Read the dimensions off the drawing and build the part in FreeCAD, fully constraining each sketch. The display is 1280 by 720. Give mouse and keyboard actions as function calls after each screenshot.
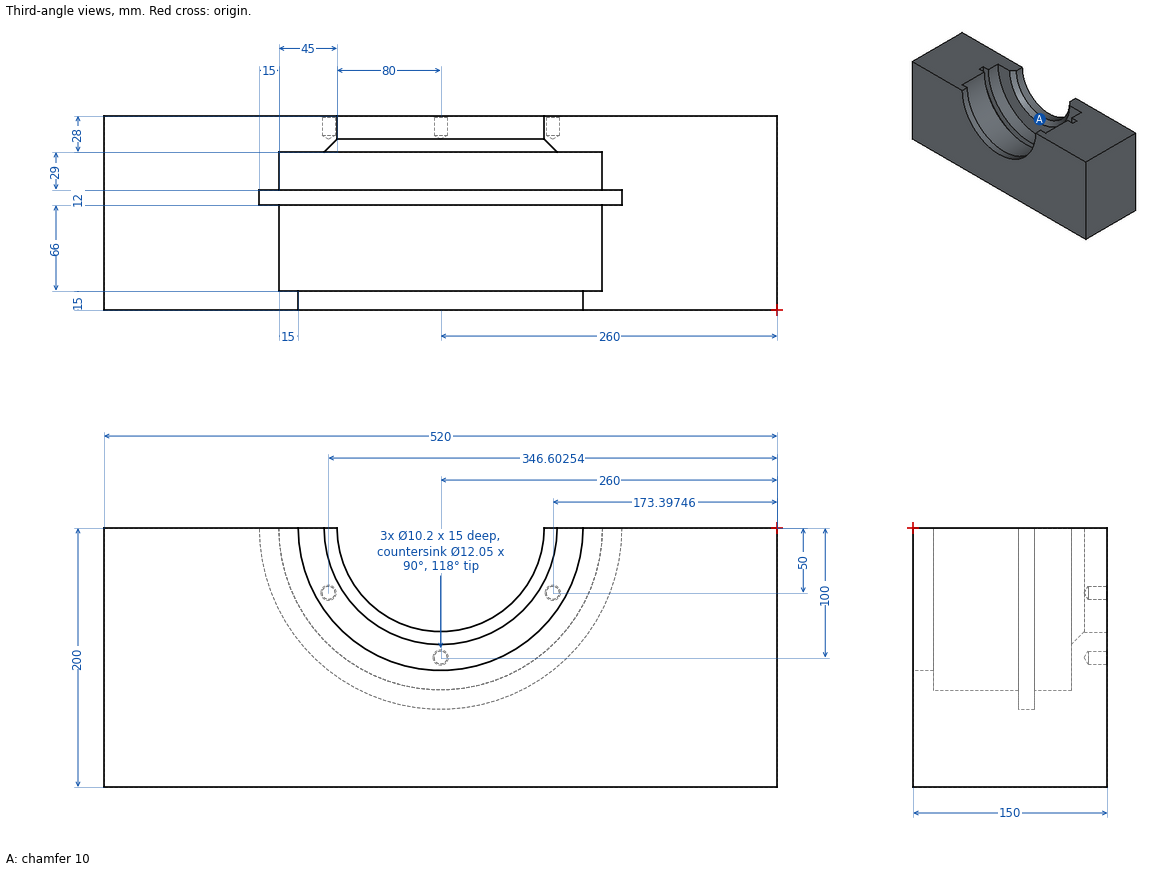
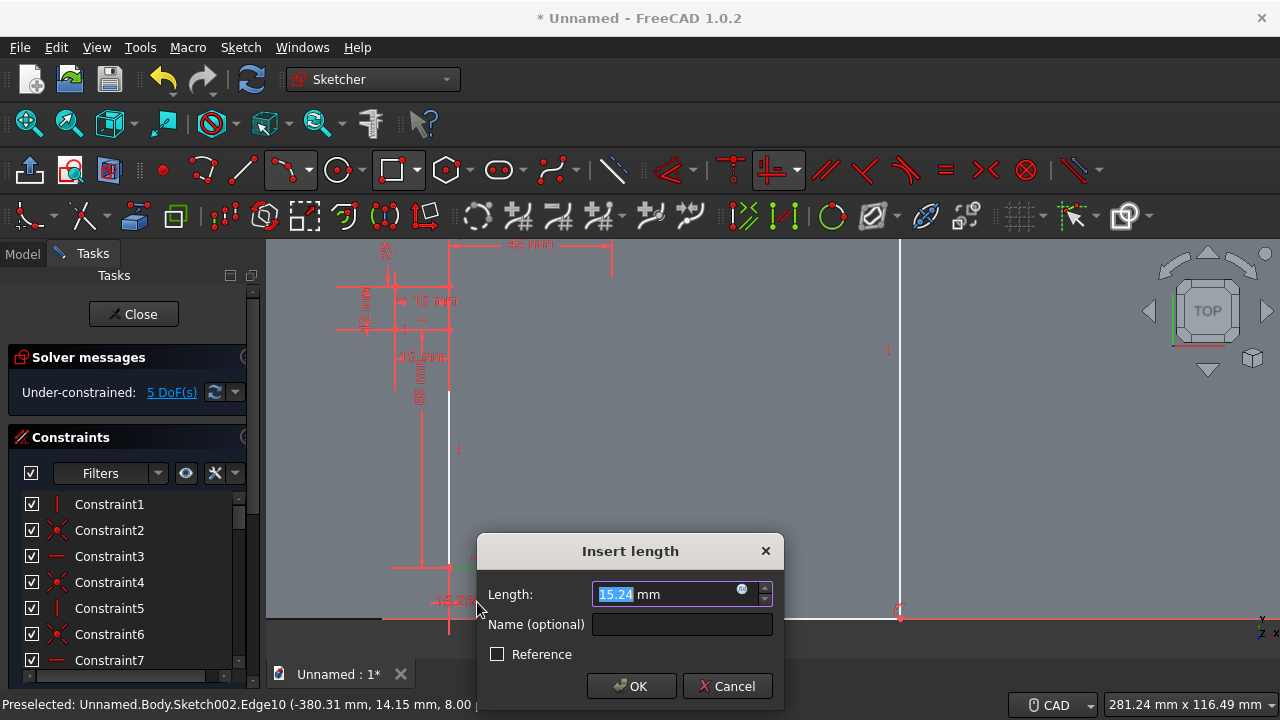
text(15)
key(Return)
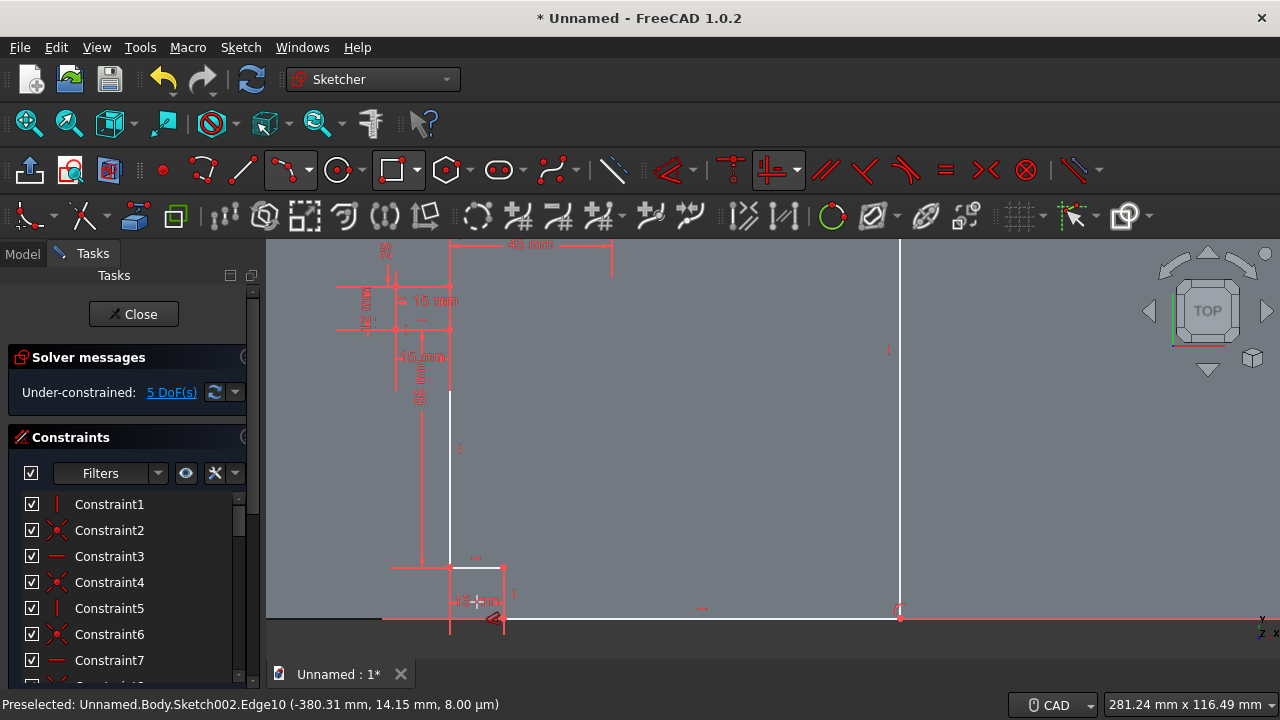
click(504, 583)
click(470, 582)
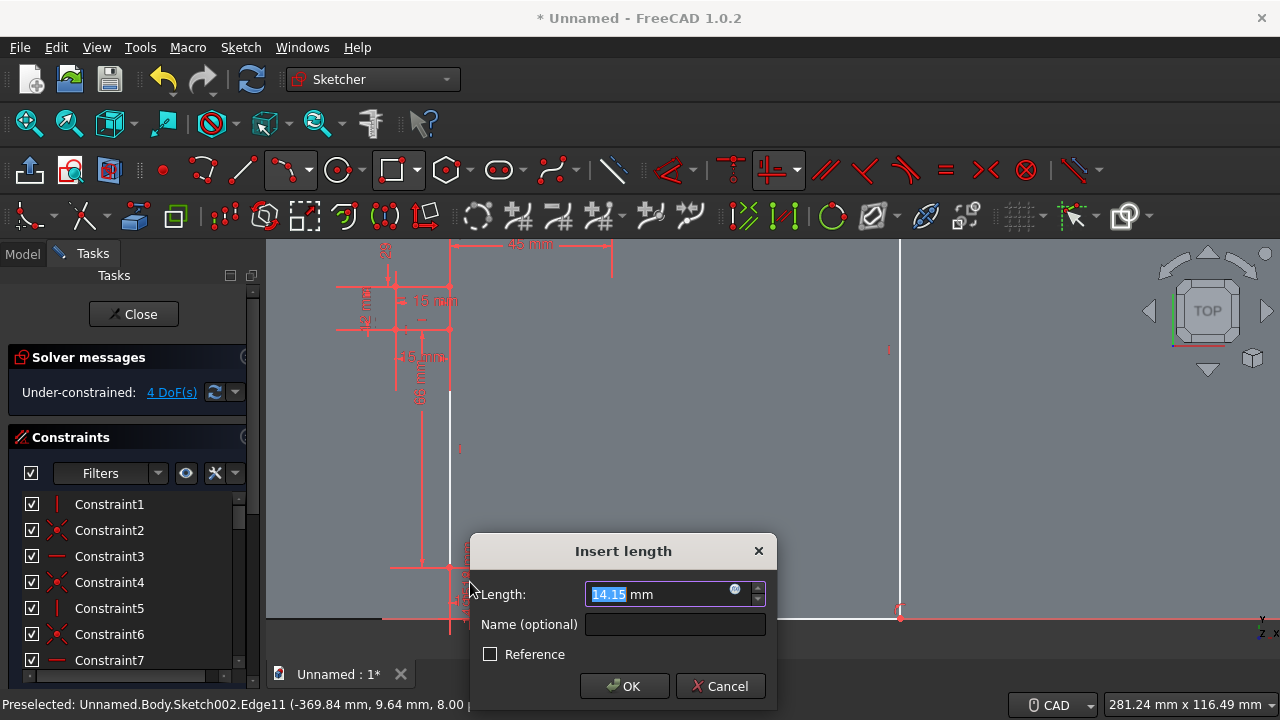
text(15)
key(Return)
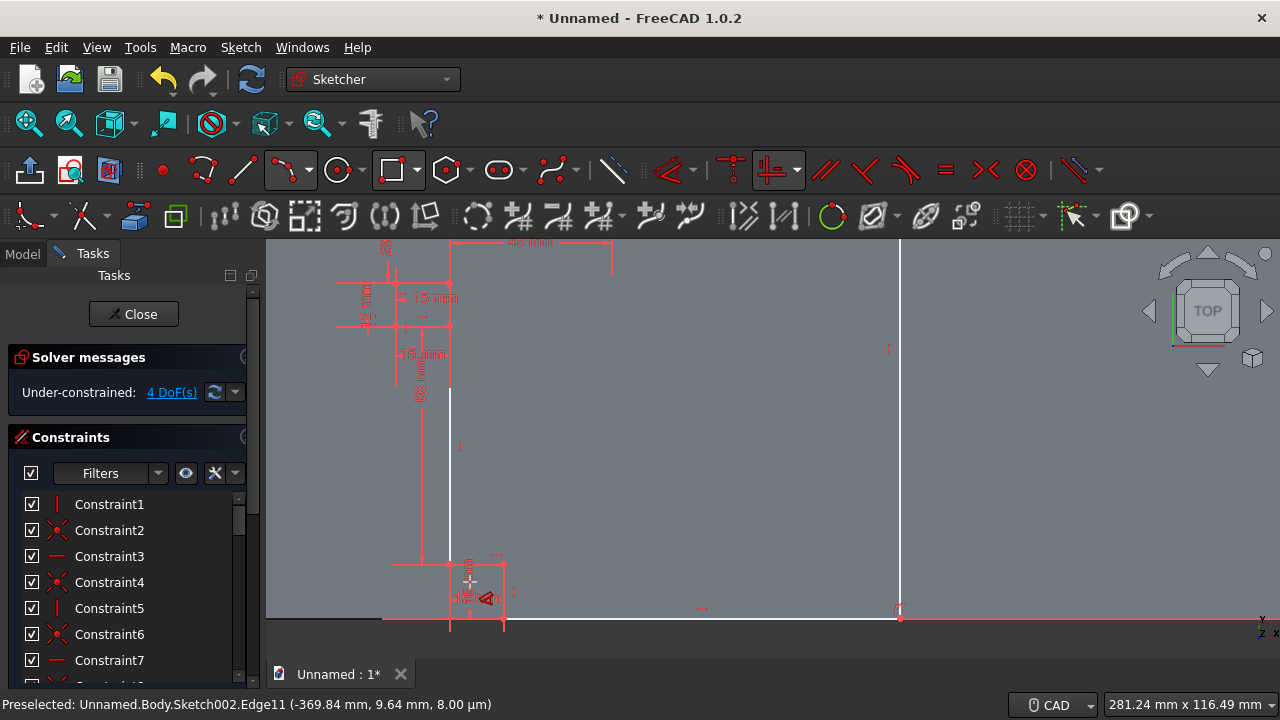
click(900, 619)
click(1008, 585)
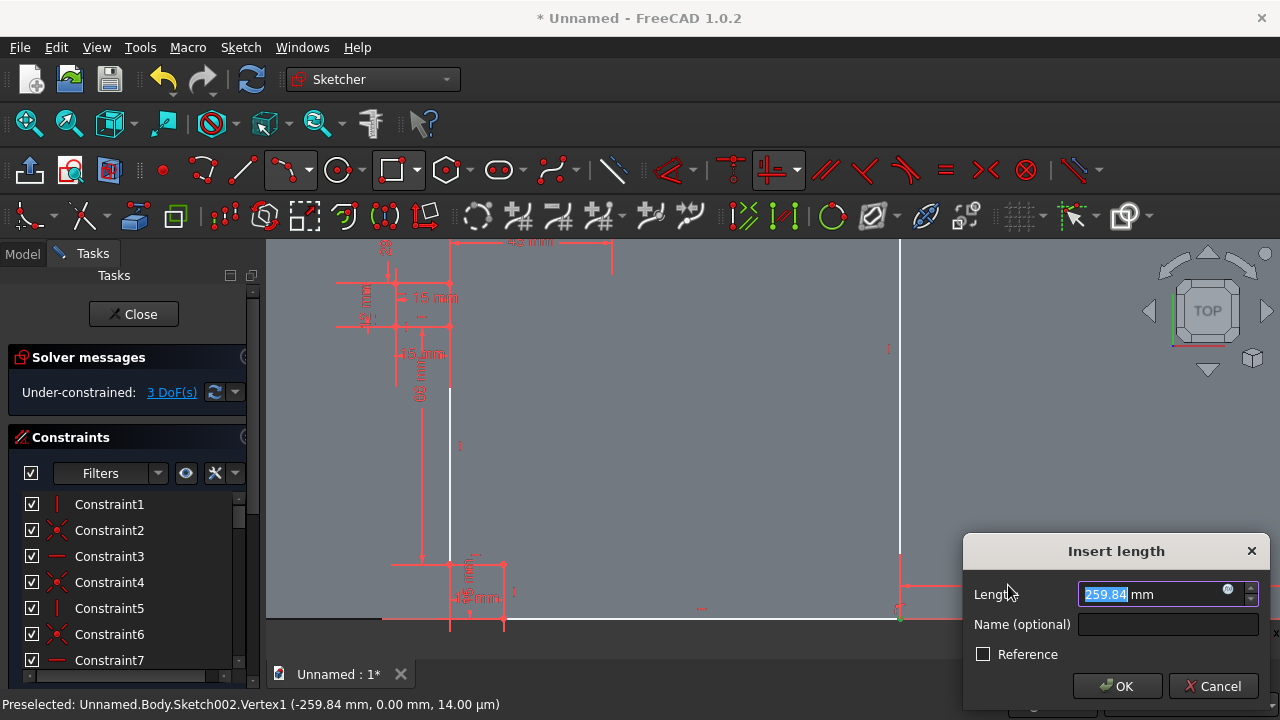
text(260)
key(Return)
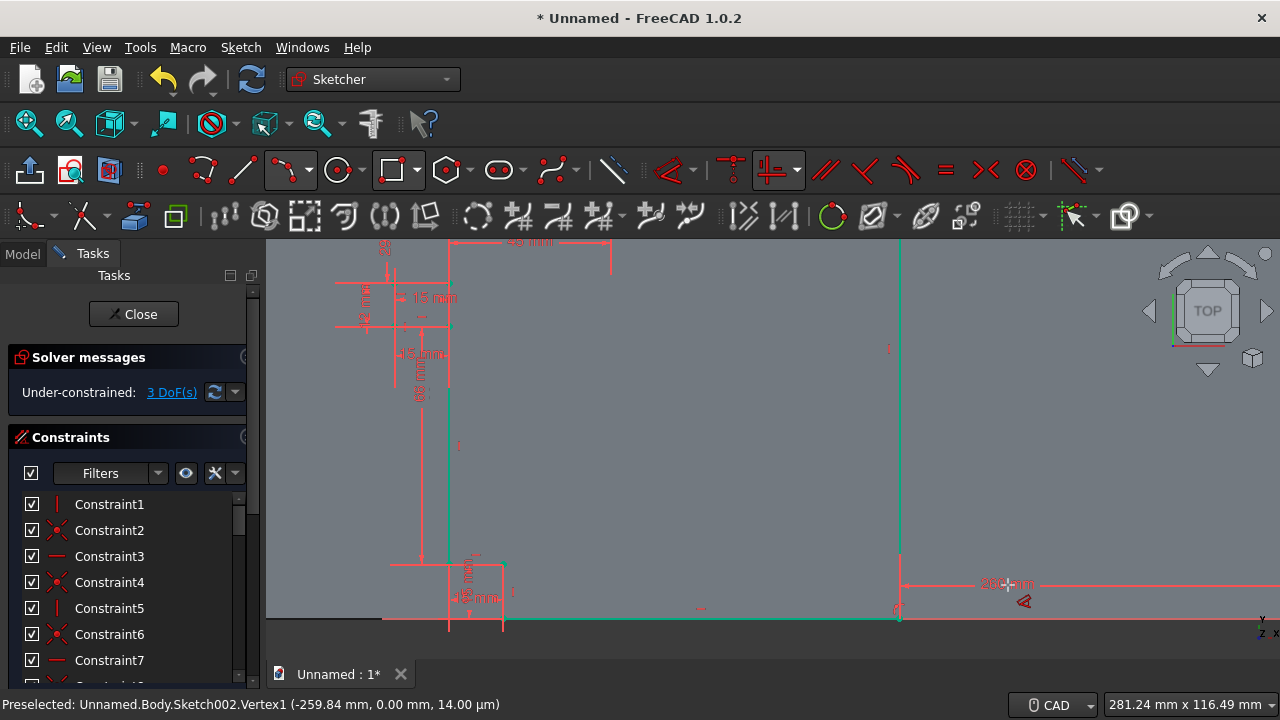
scroll(465, 571, down, 5)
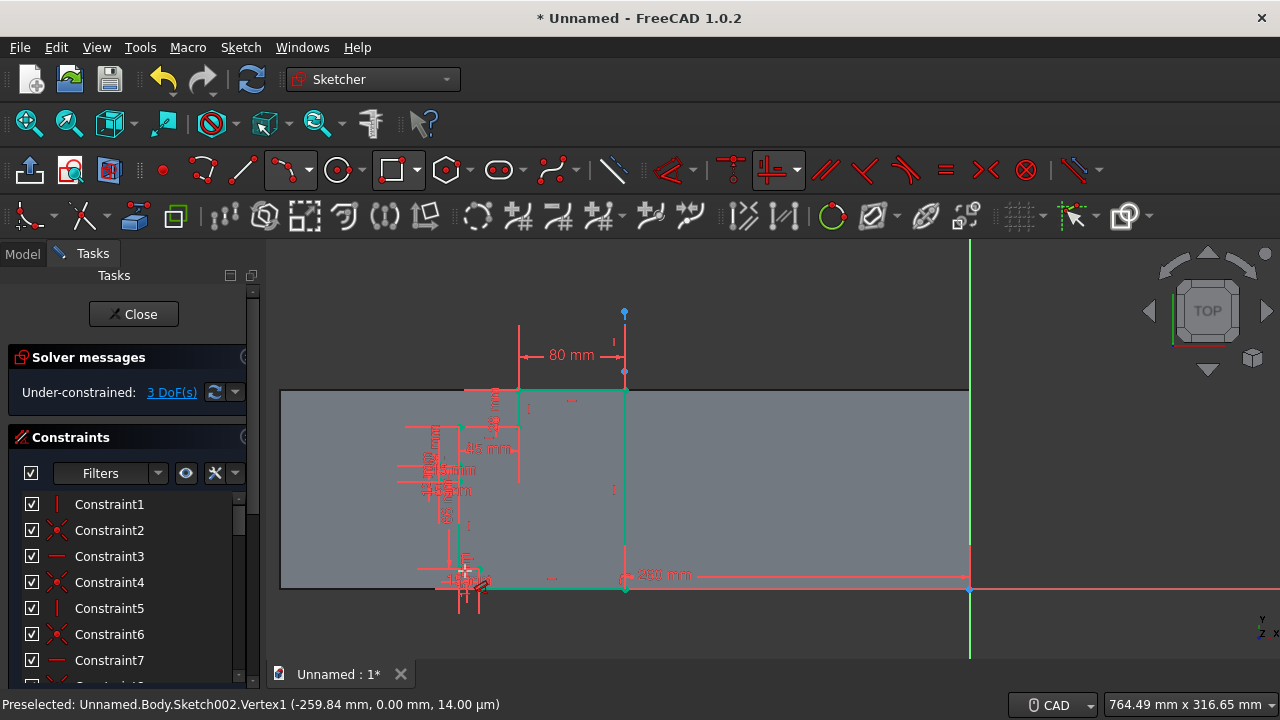
click(625, 371)
click(797, 623)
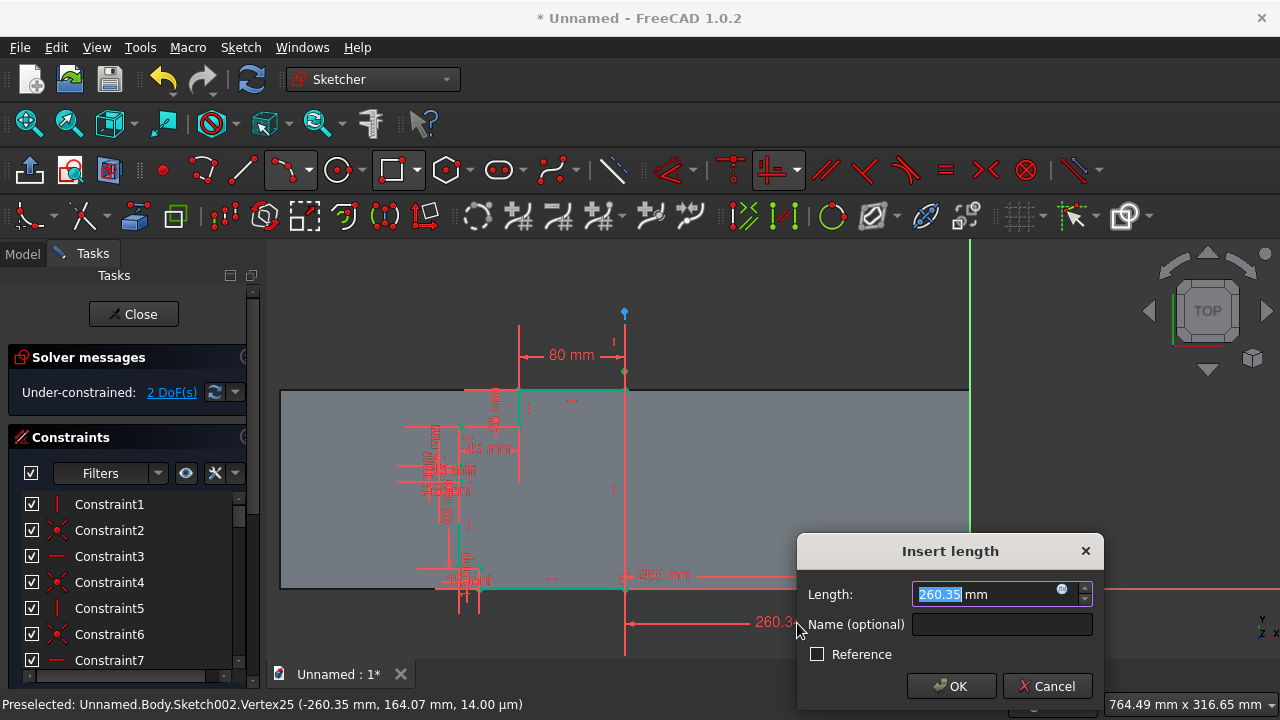
text(260)
key(Return)
key(Escape)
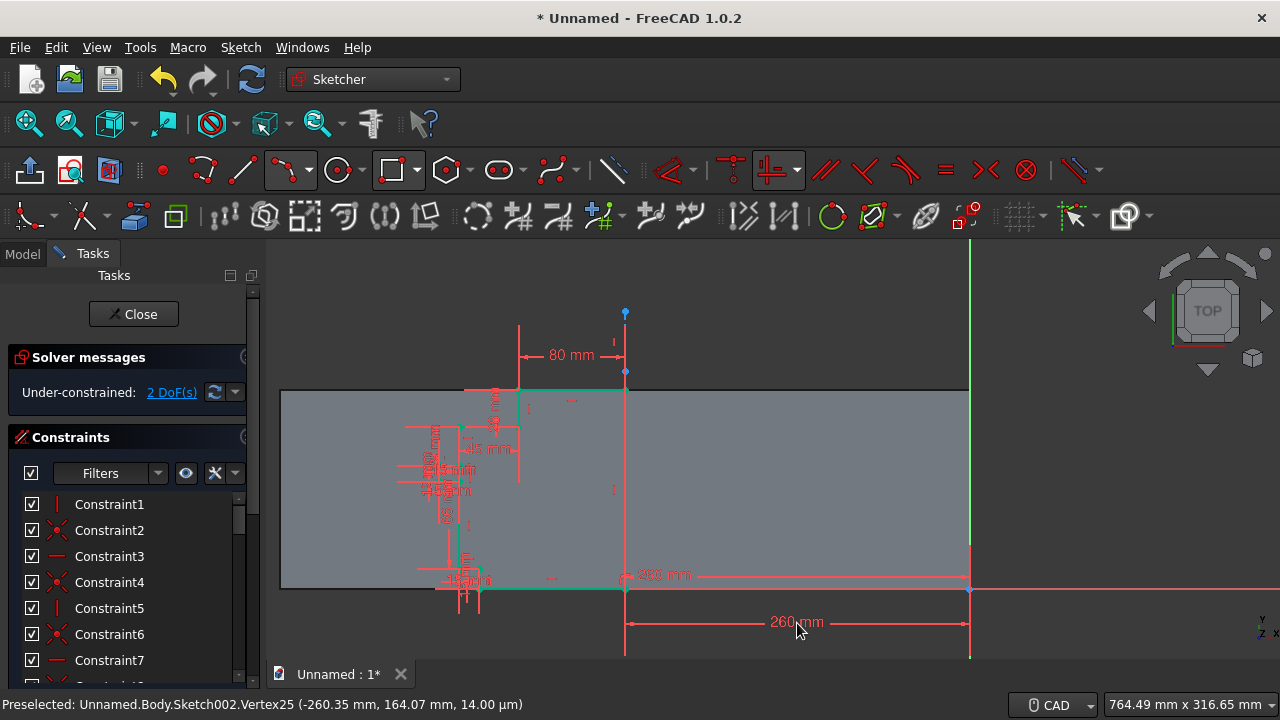
click(134, 314)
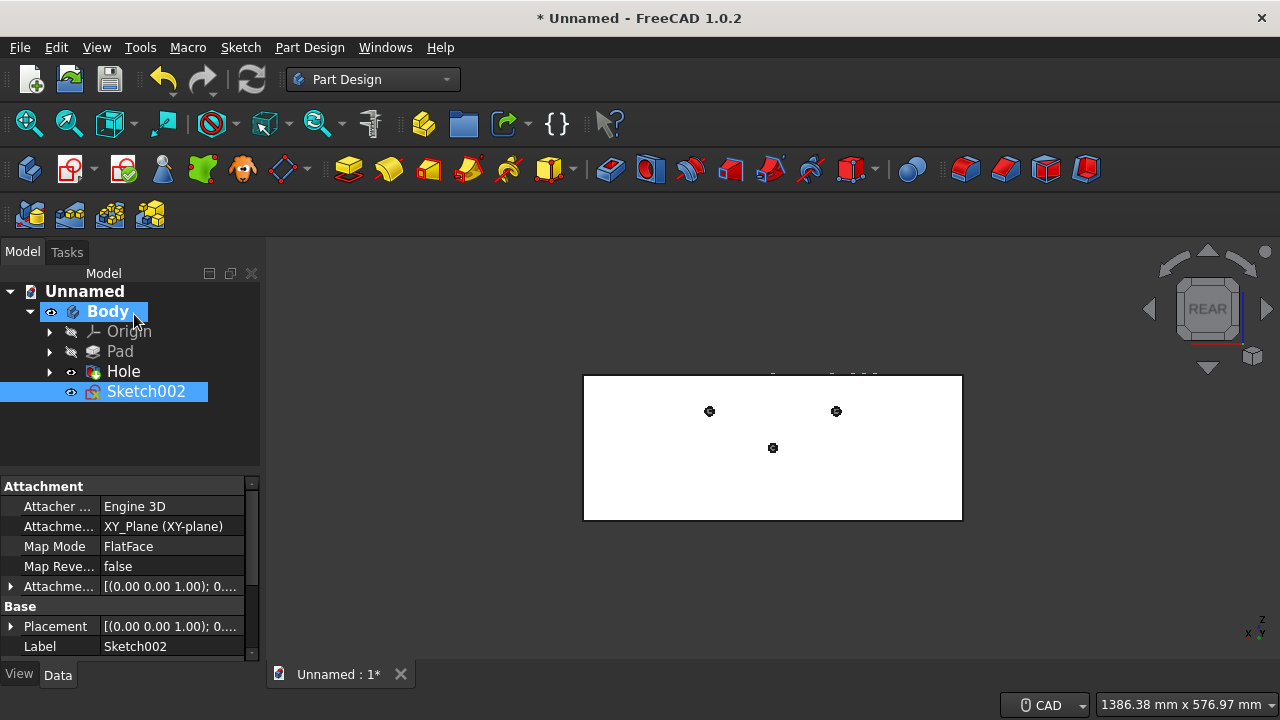
click(692, 170)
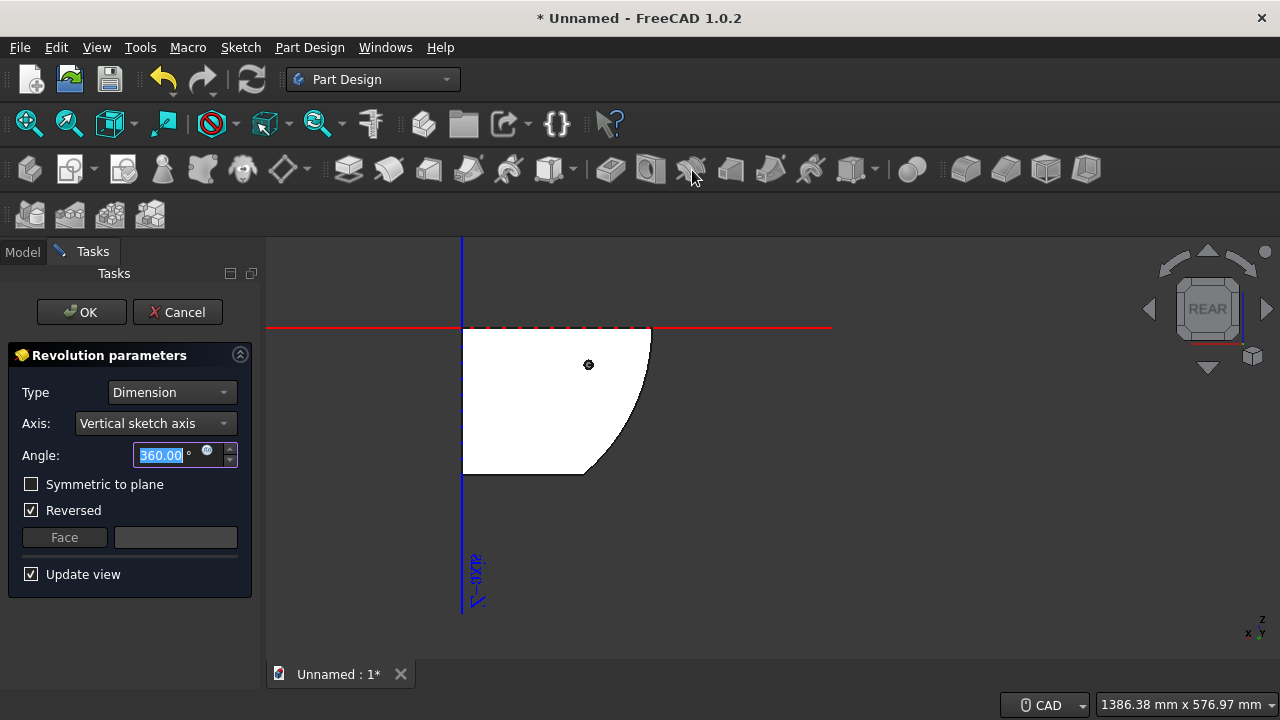
click(156, 424)